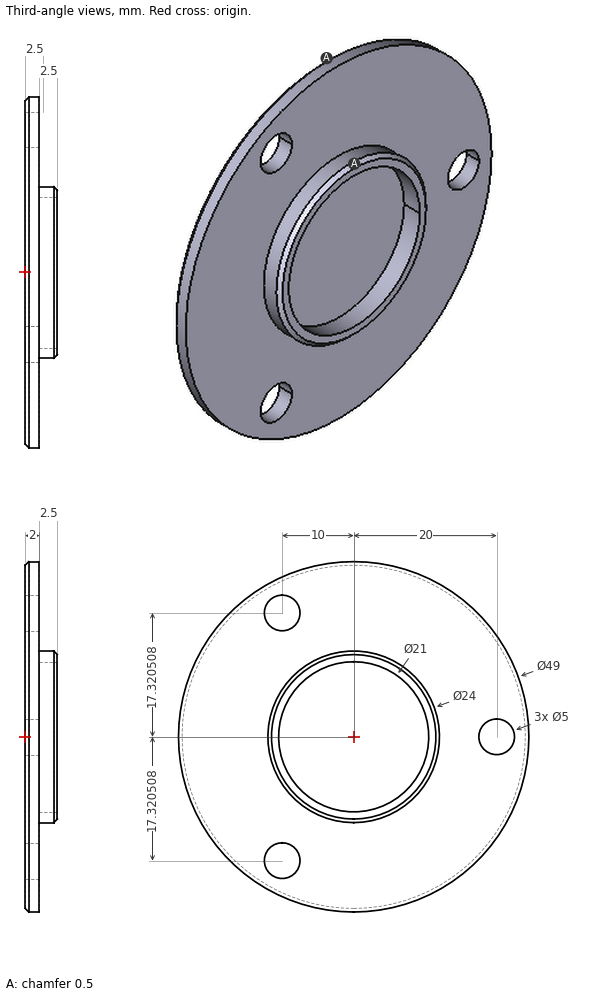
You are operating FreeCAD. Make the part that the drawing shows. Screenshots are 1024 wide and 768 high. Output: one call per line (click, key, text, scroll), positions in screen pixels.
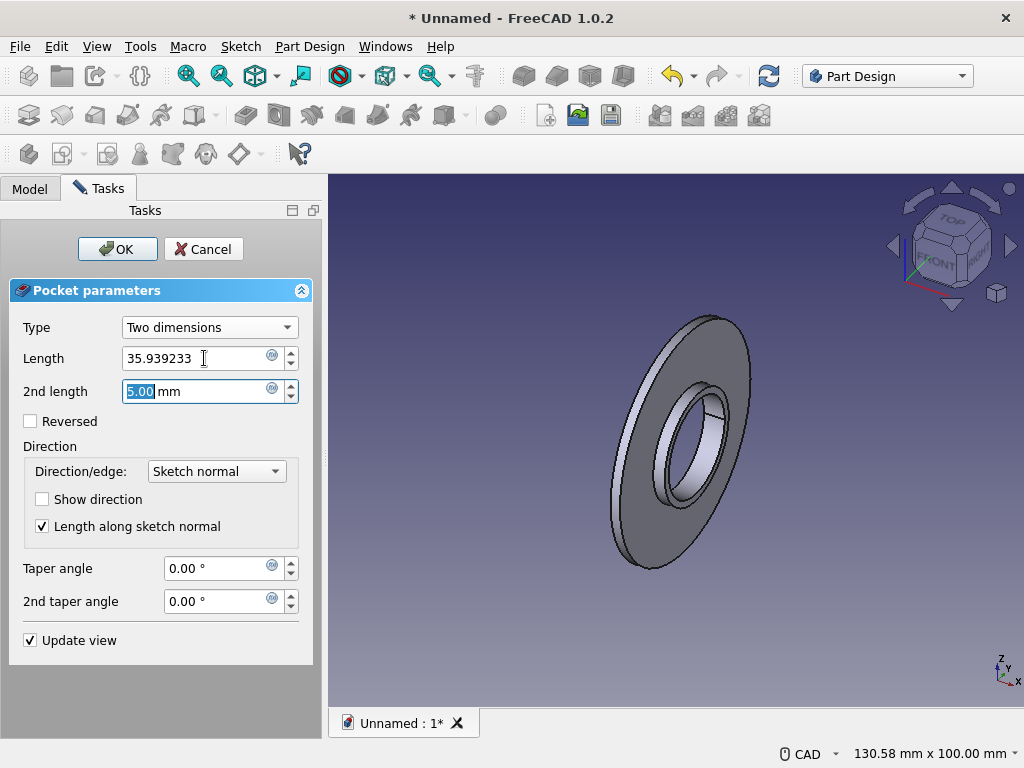
text(2.5)
key(Tab)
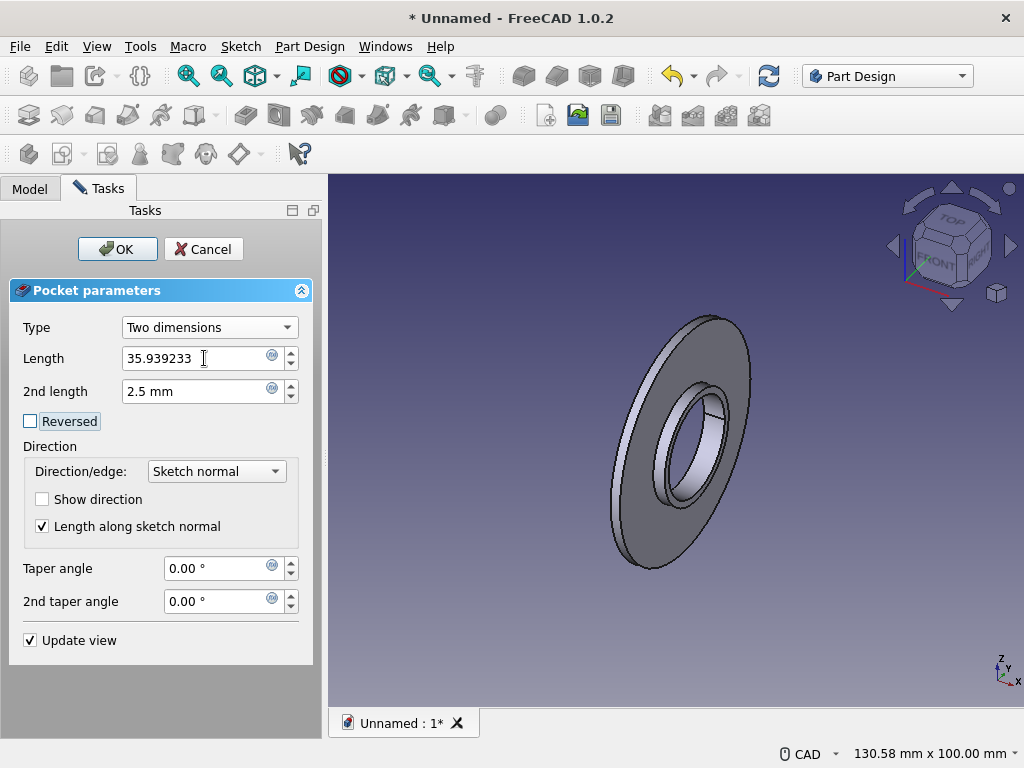
click(31, 421)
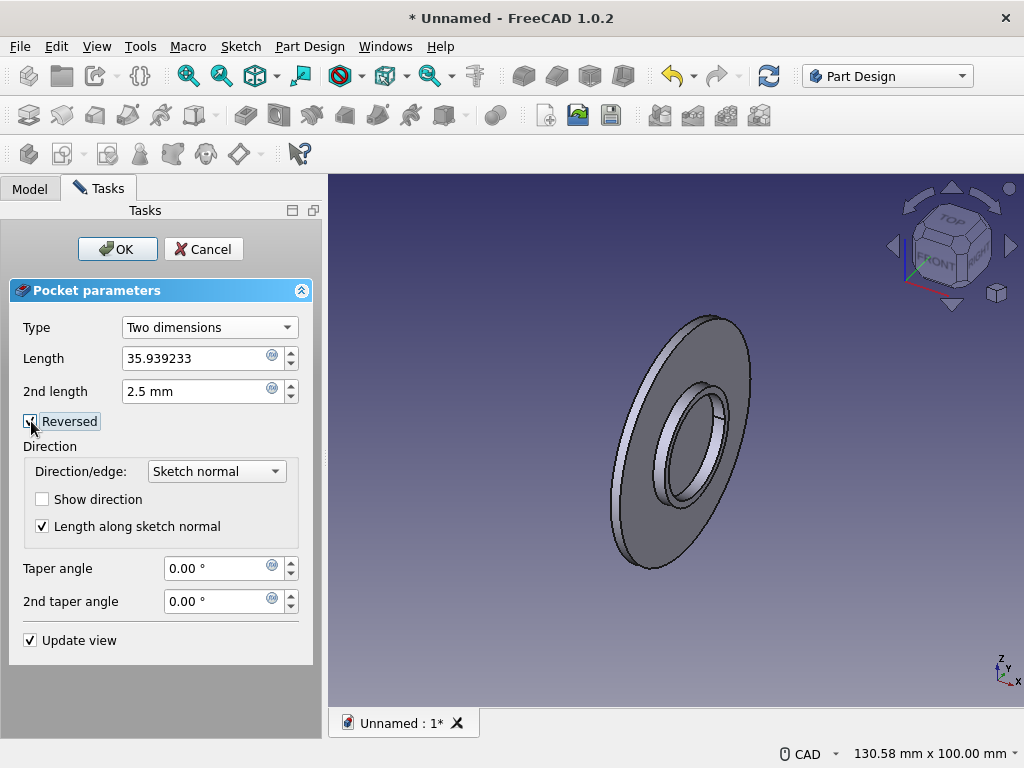
click(118, 249)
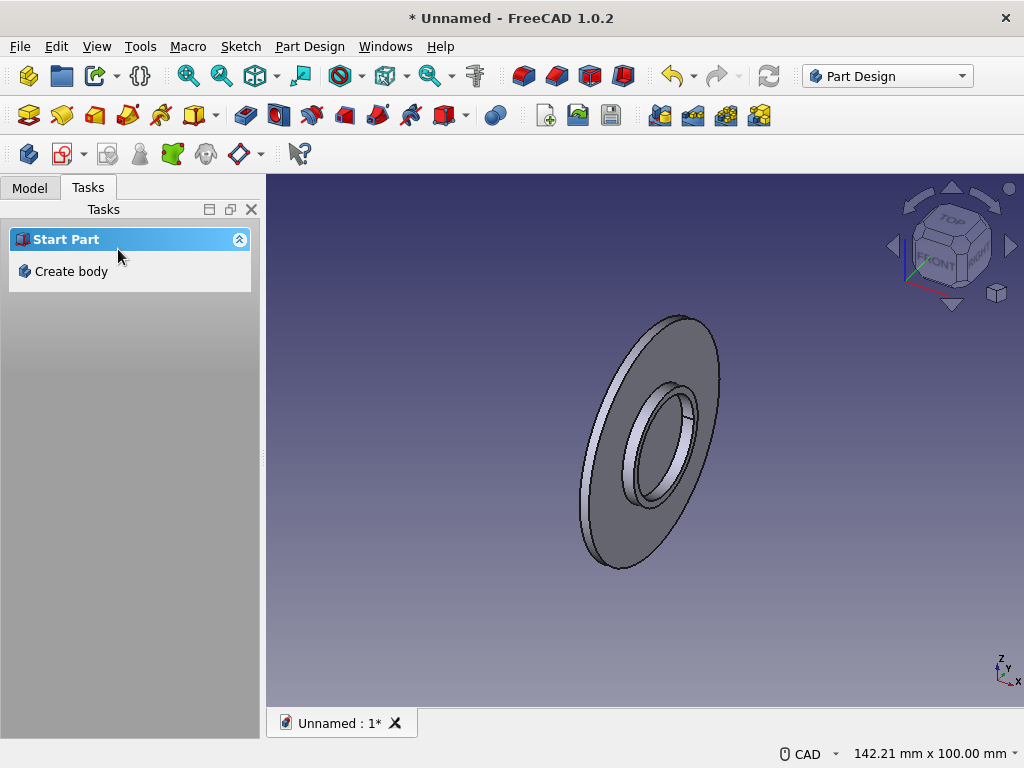
key(6)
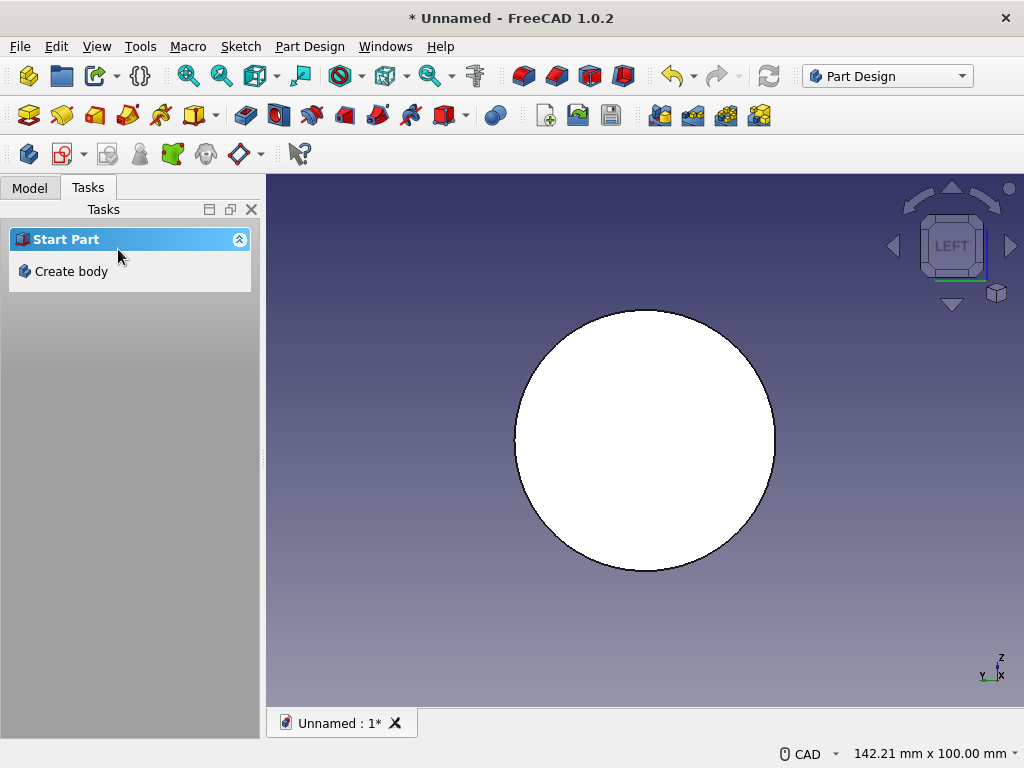
click(645, 439)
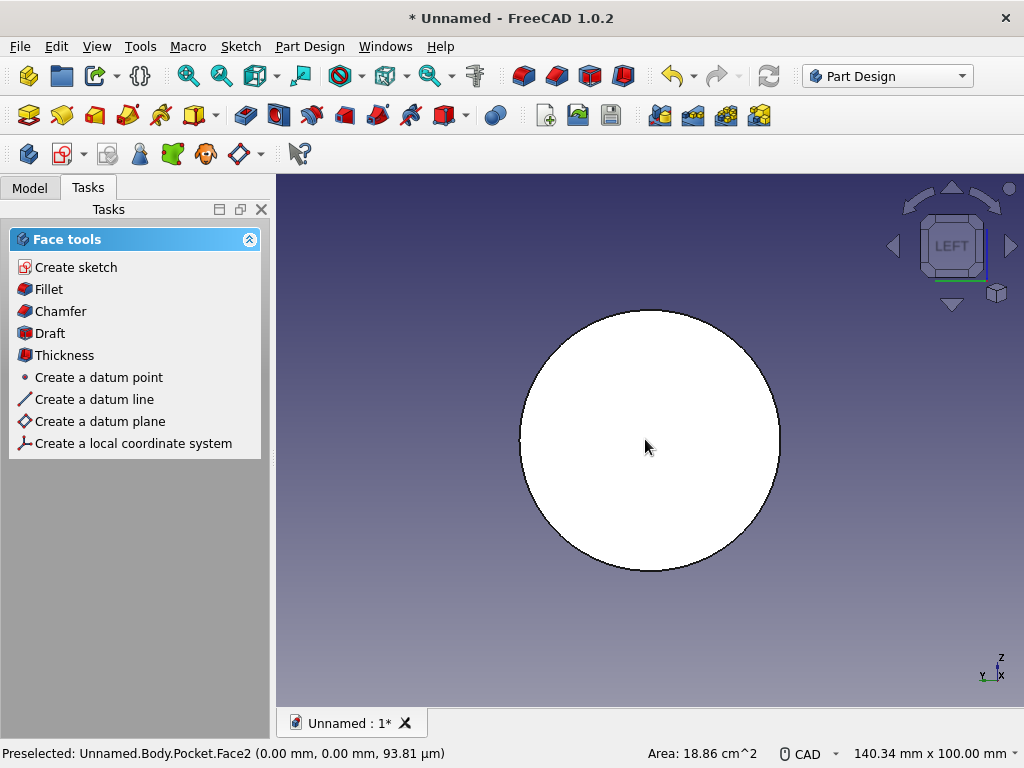
click(62, 154)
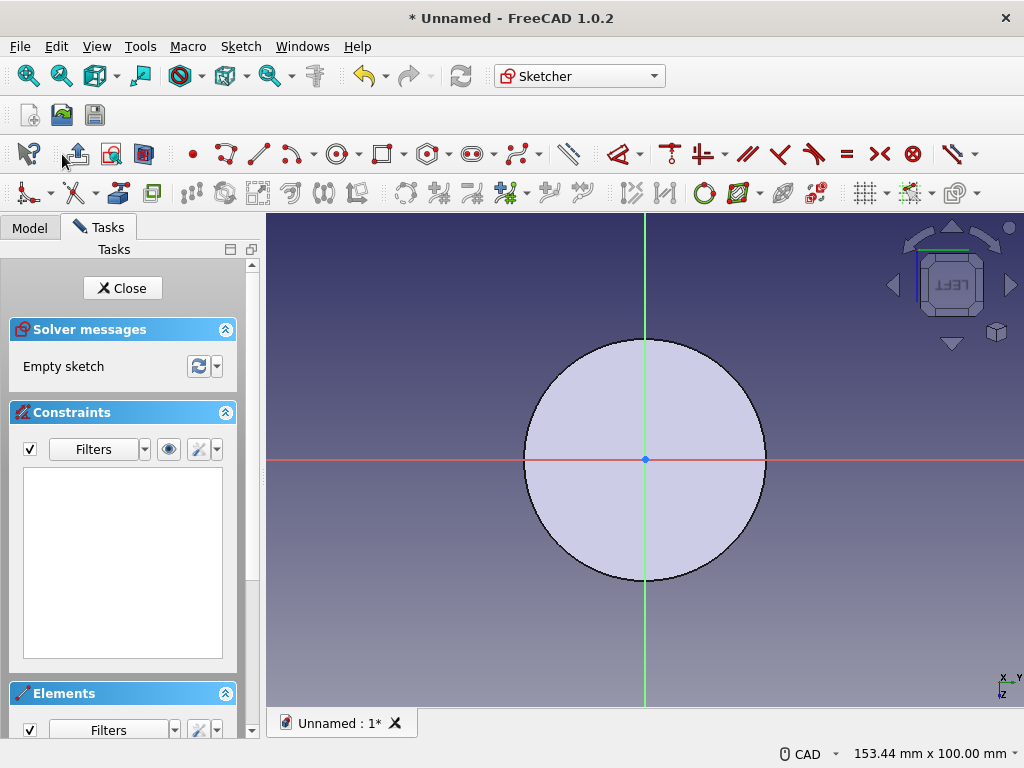
scroll(859, 460, up, 2)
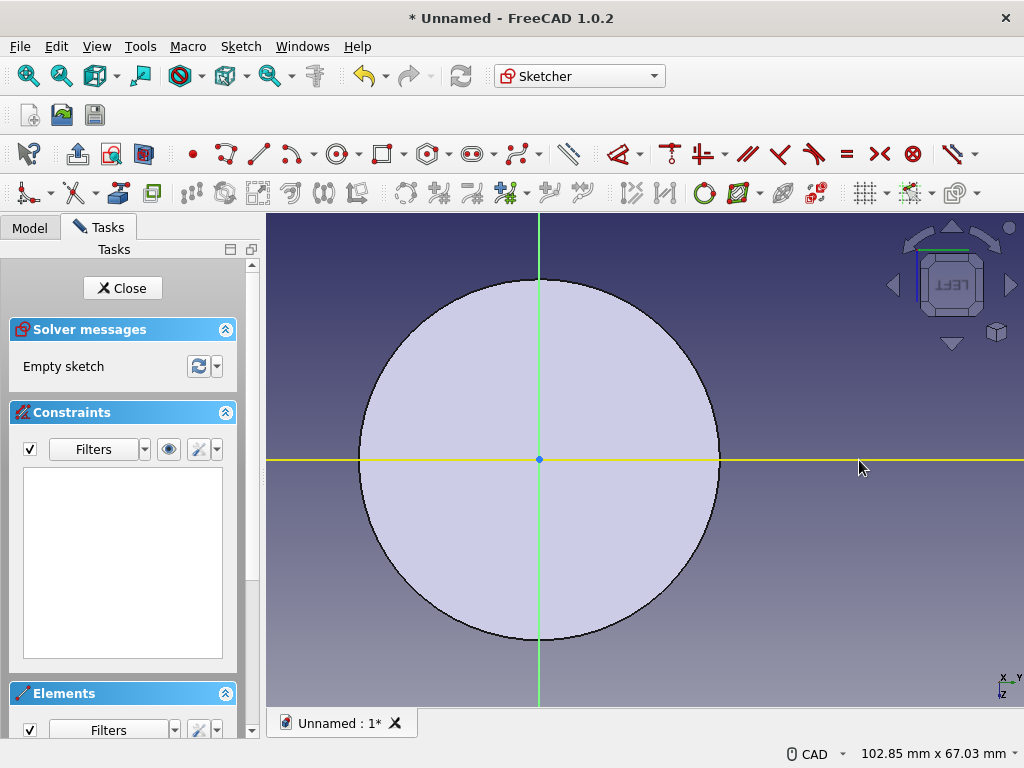
click(336, 154)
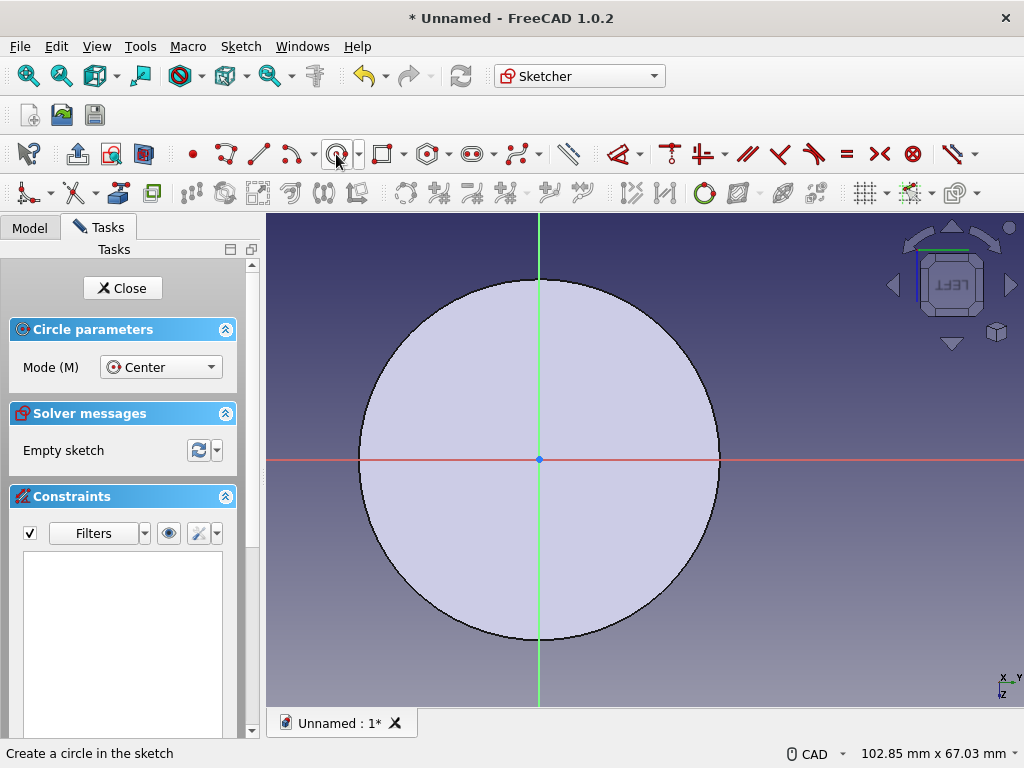
scroll(687, 460, up, 2)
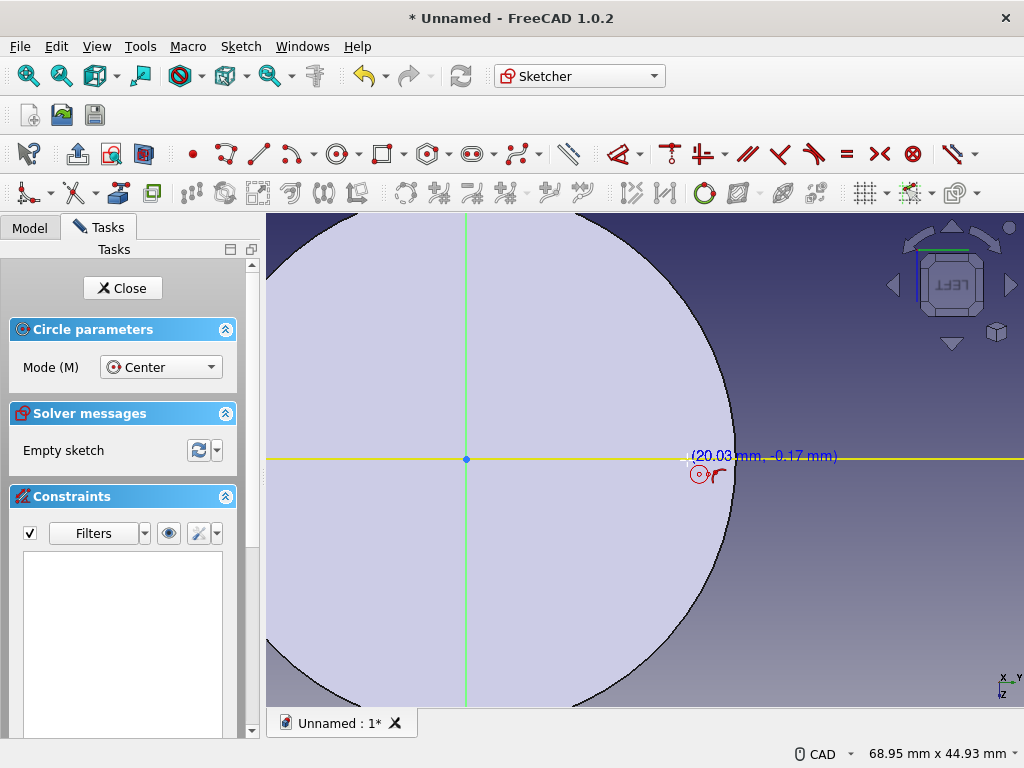
click(686, 459)
click(706, 440)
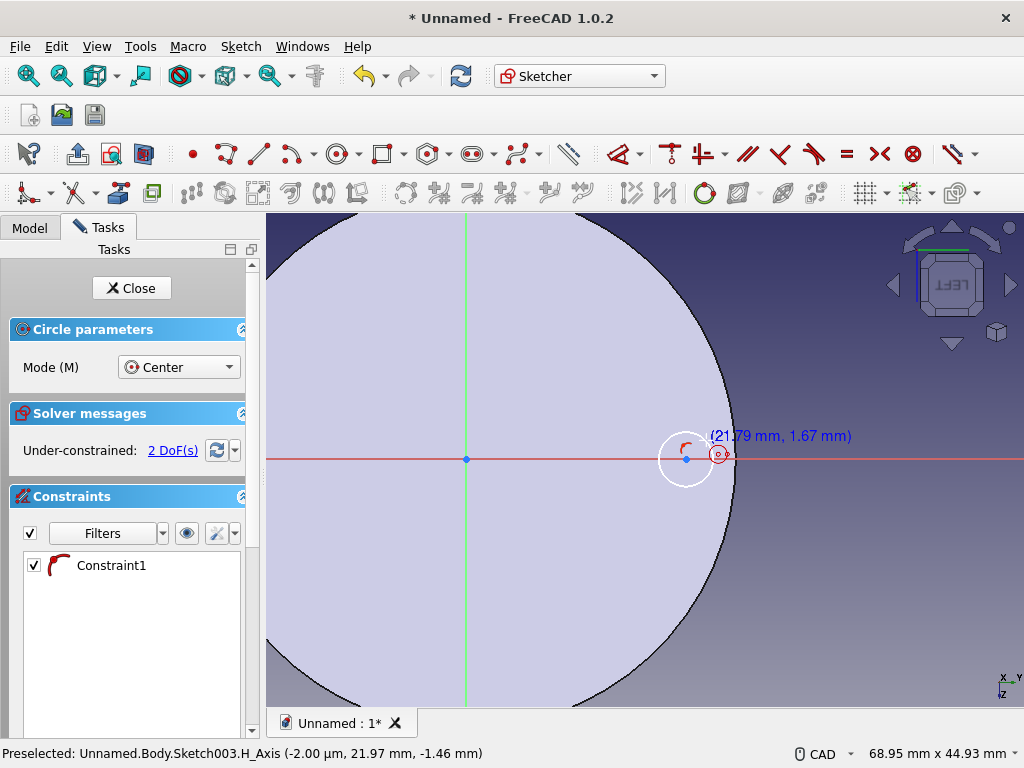
click(357, 650)
click(376, 630)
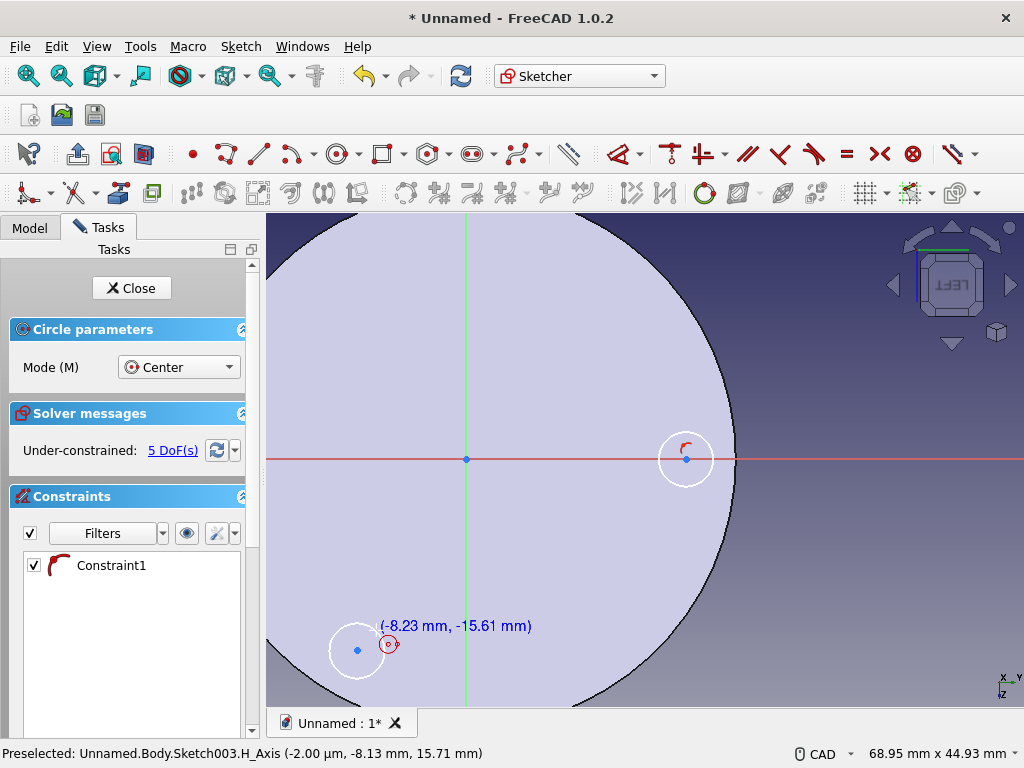
click(357, 269)
click(376, 250)
key(Escape)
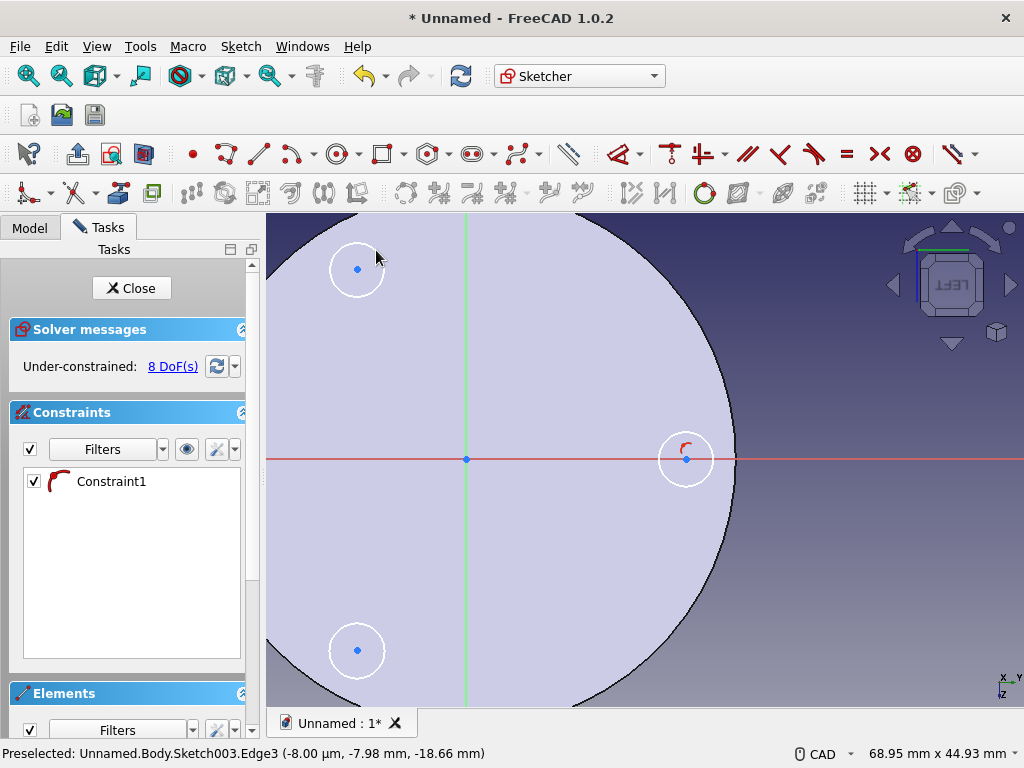
click(705, 440)